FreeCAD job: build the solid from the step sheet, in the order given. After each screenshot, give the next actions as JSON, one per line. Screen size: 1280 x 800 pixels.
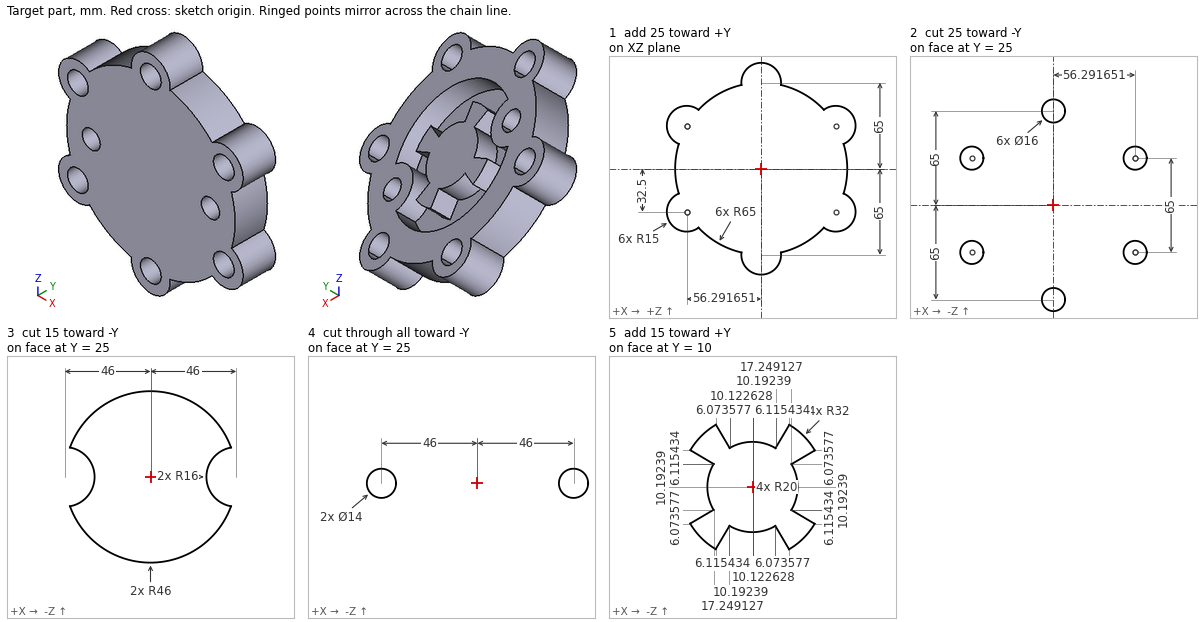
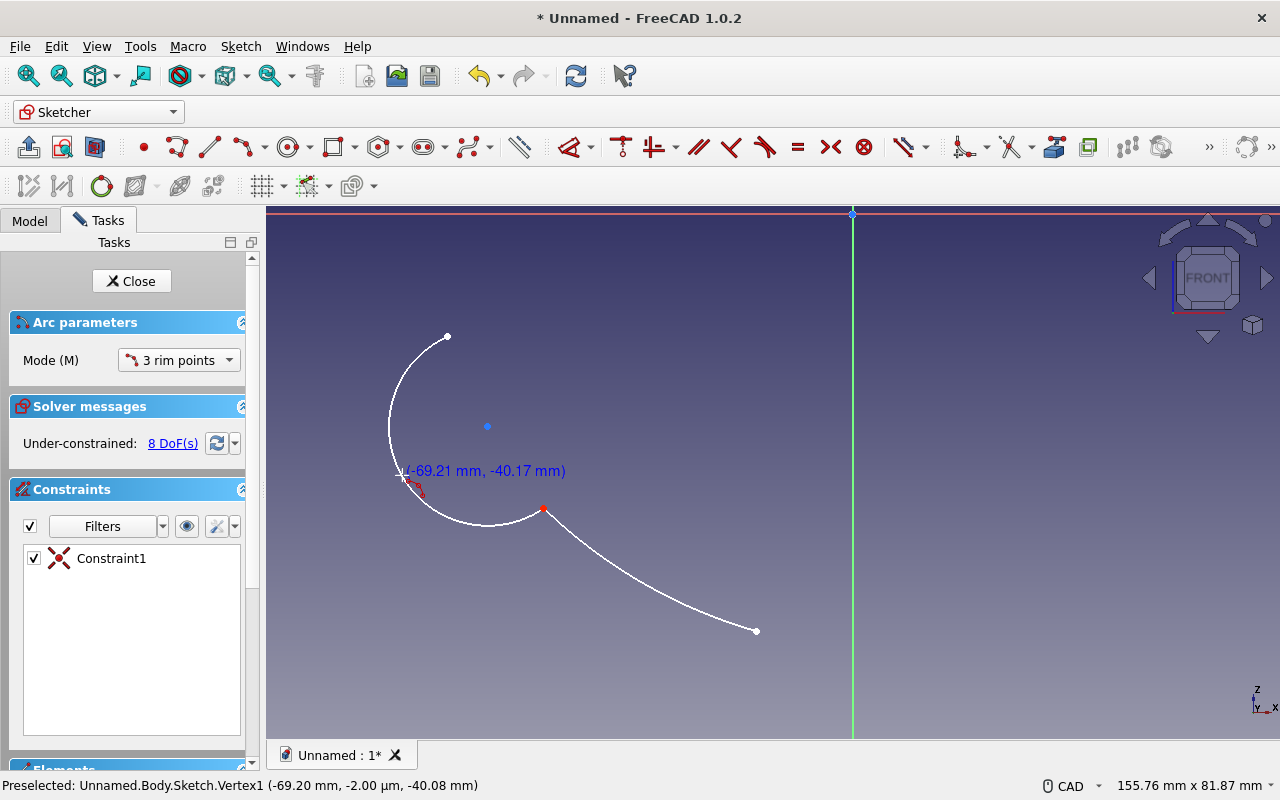
{"action": "left_click", "coordinate": [447, 337]}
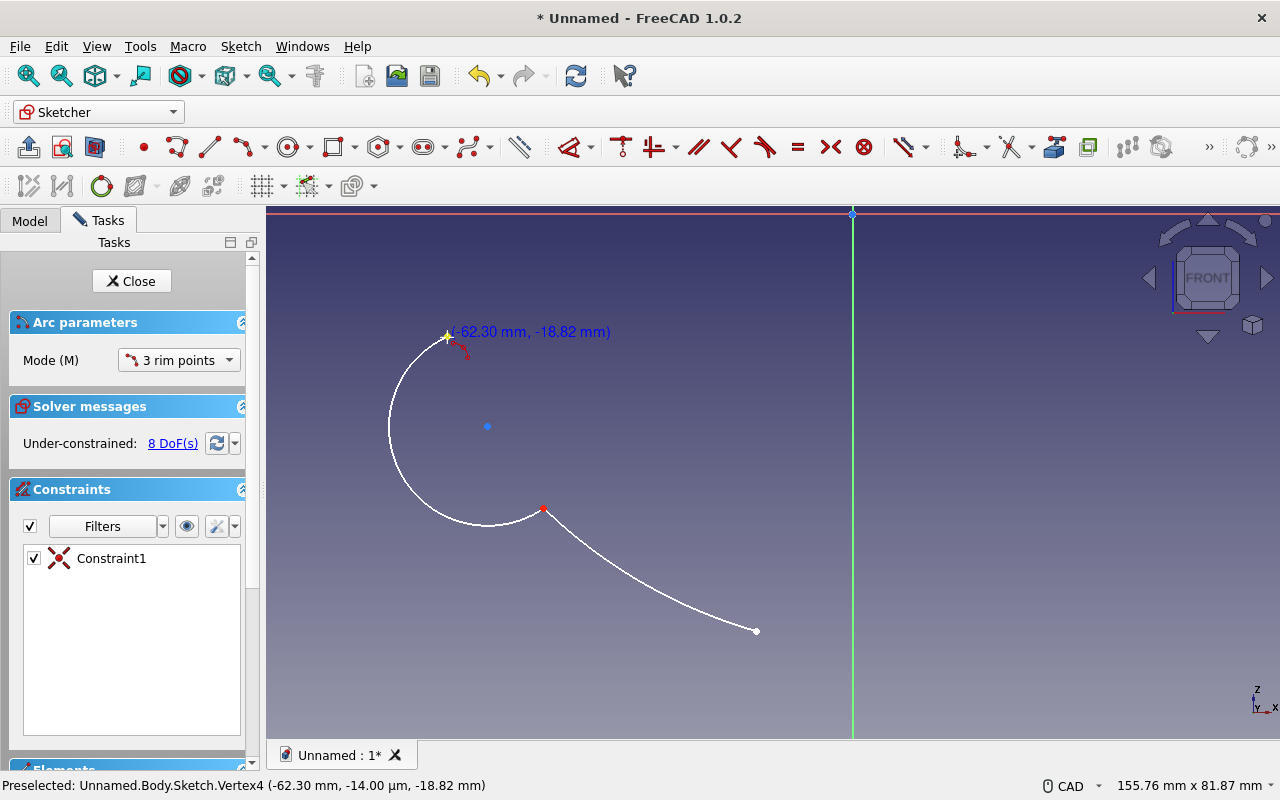
{"action": "scroll", "coordinate": [641, 584], "scroll_direction": "down", "scroll_amount": 6}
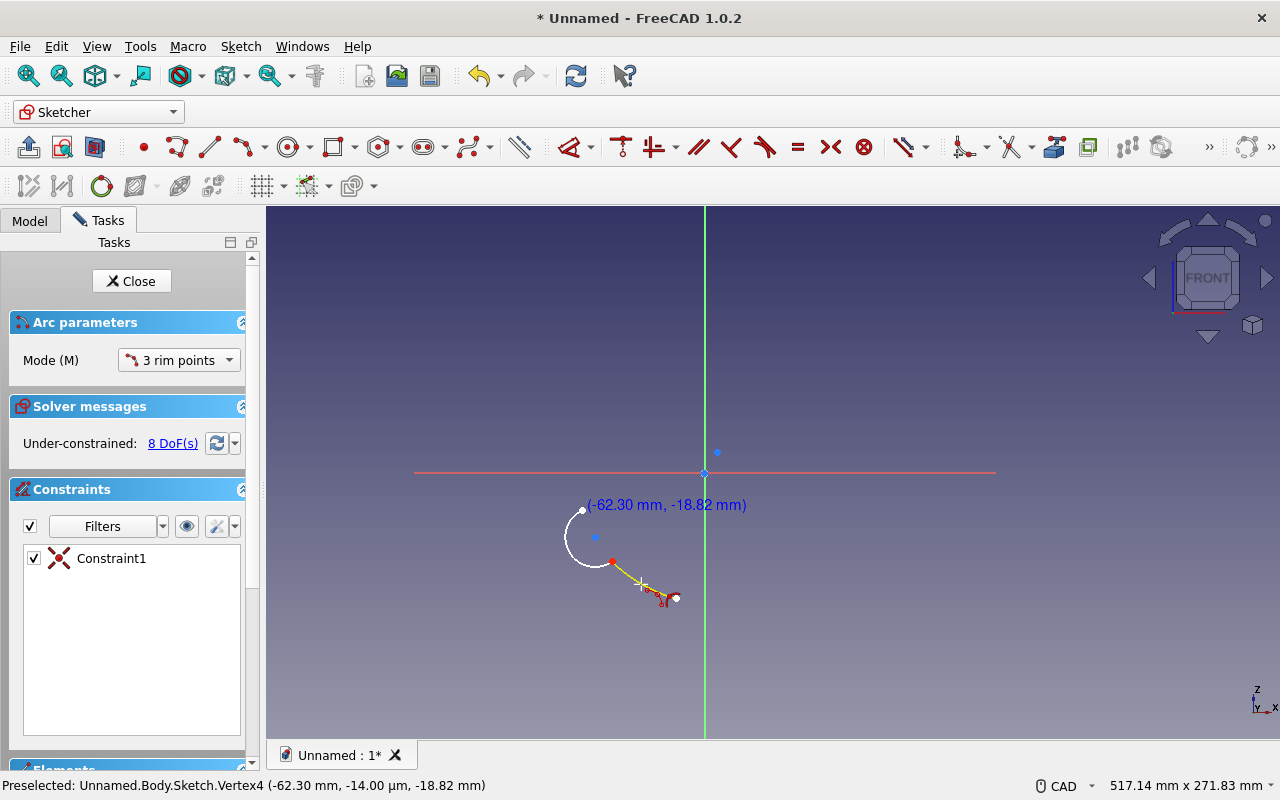
{"action": "left_click", "coordinate": [583, 436]}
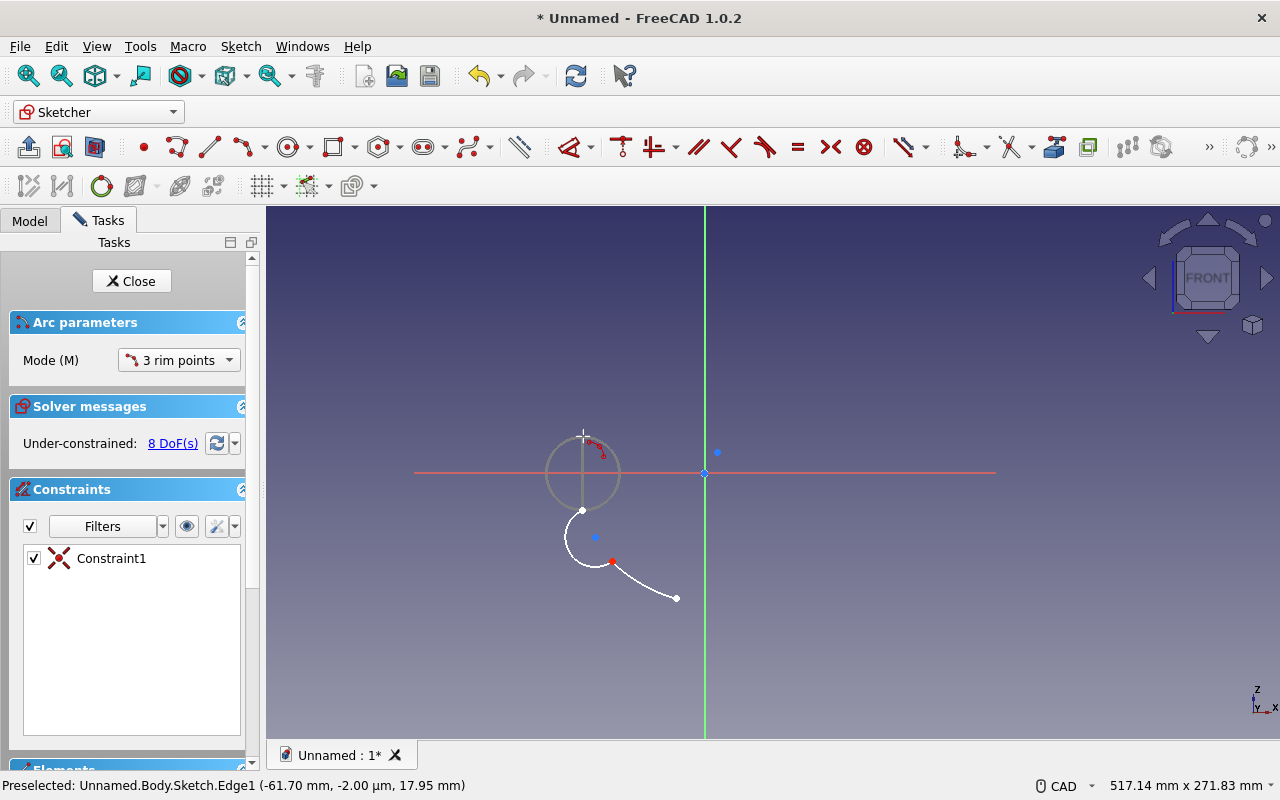
{"action": "scroll", "coordinate": [578, 466], "scroll_direction": "up", "scroll_amount": 6}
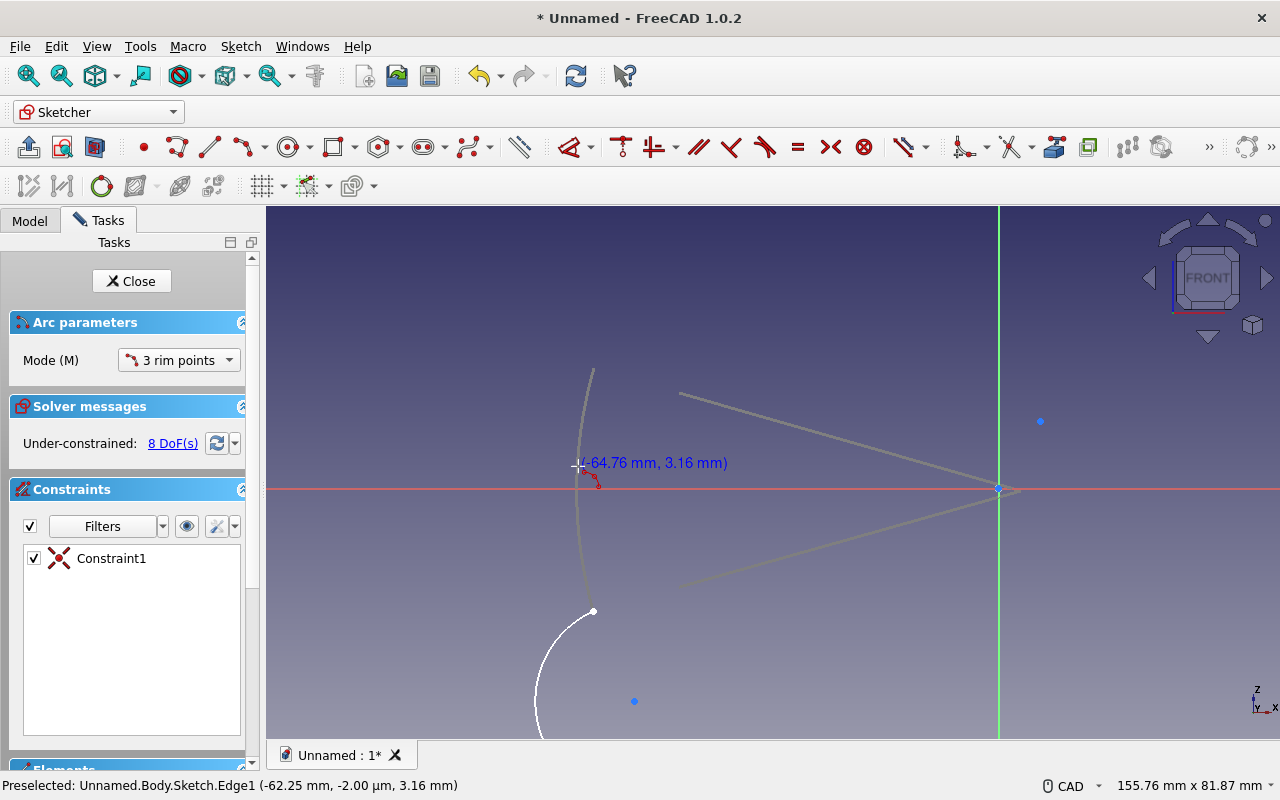
{"action": "left_click", "coordinate": [576, 464]}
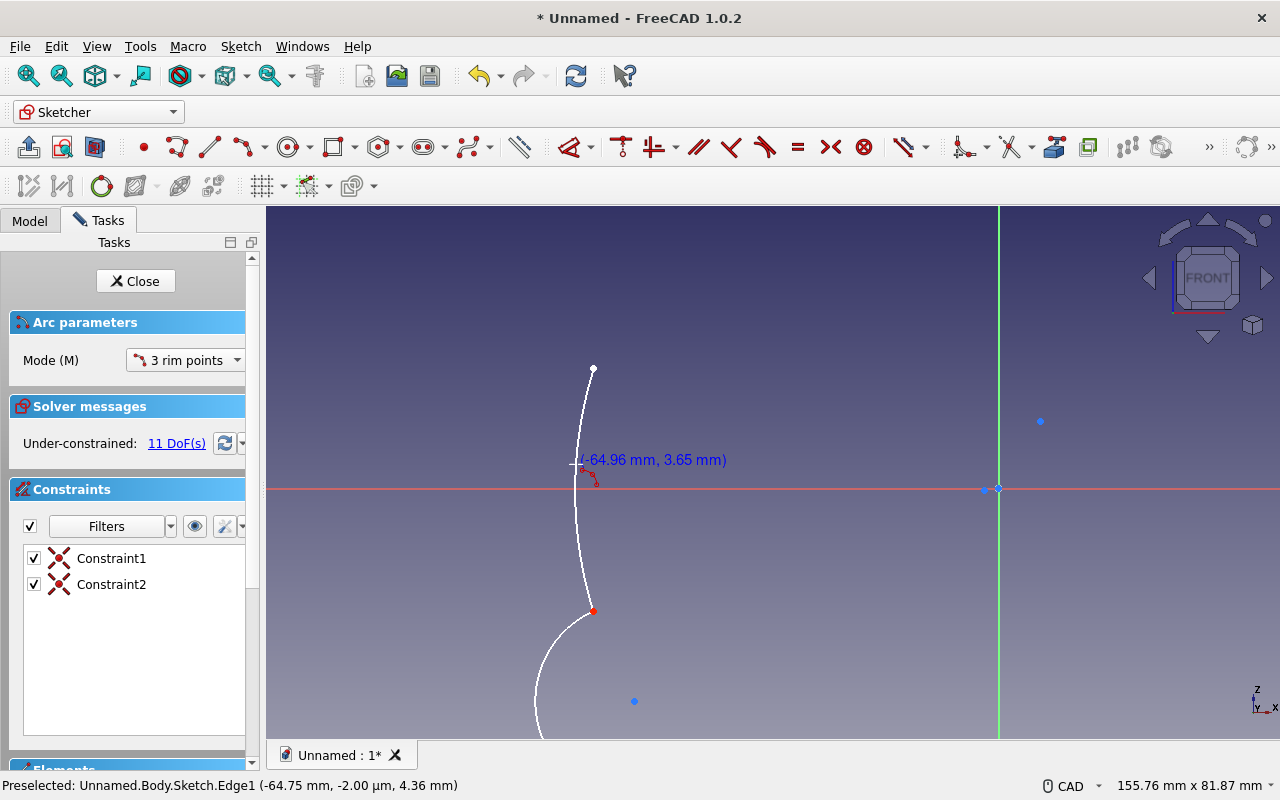
{"action": "left_click", "coordinate": [594, 369]}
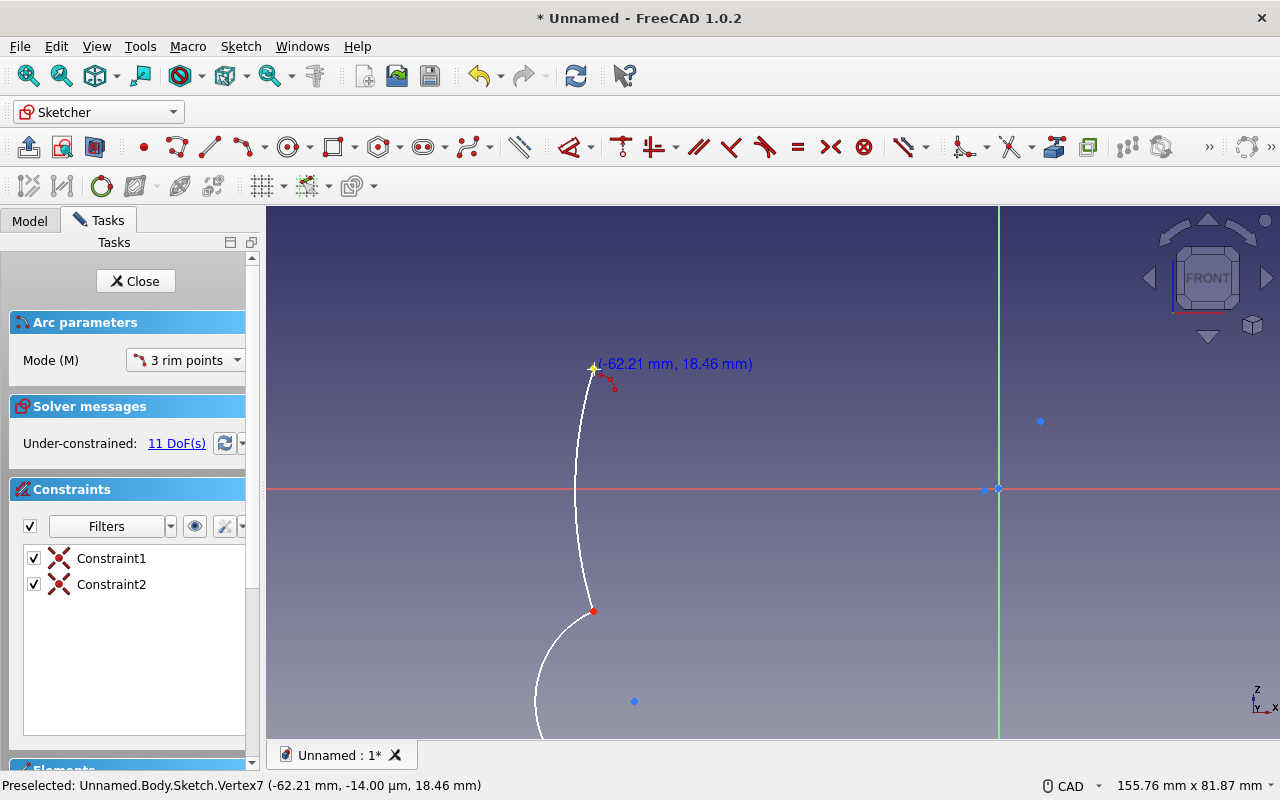
{"action": "scroll", "coordinate": [578, 465], "scroll_direction": "down", "scroll_amount": 6}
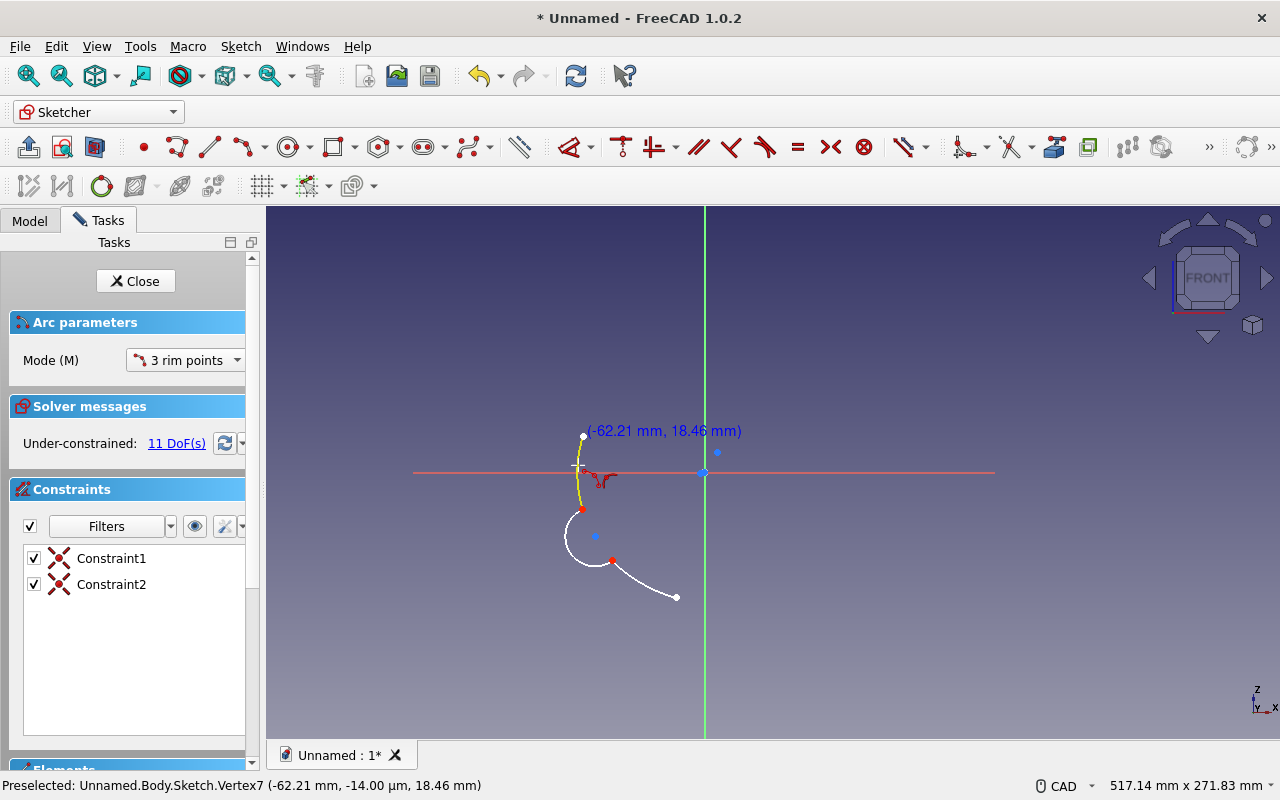
{"action": "left_click", "coordinate": [612, 385]}
{"action": "left_click", "coordinate": [569, 394]}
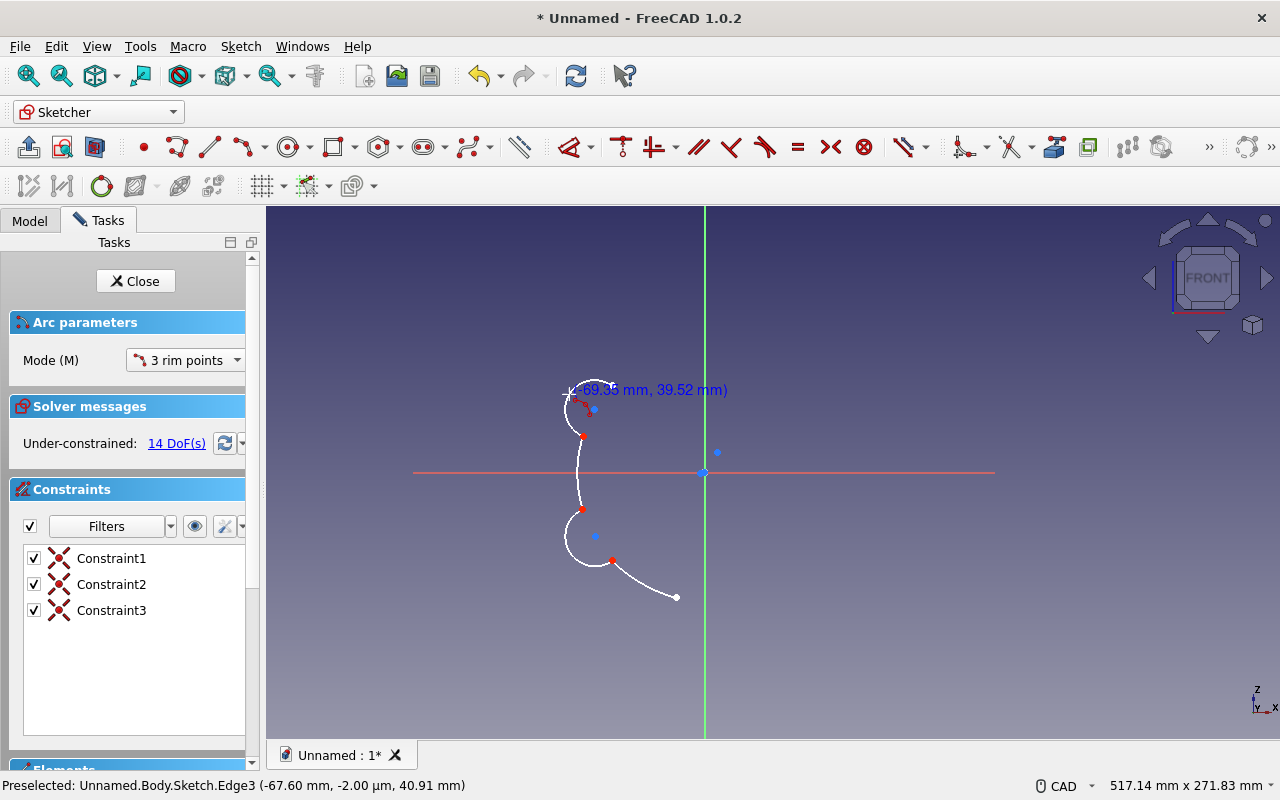
{"action": "left_click", "coordinate": [612, 386]}
{"action": "left_click", "coordinate": [676, 348]}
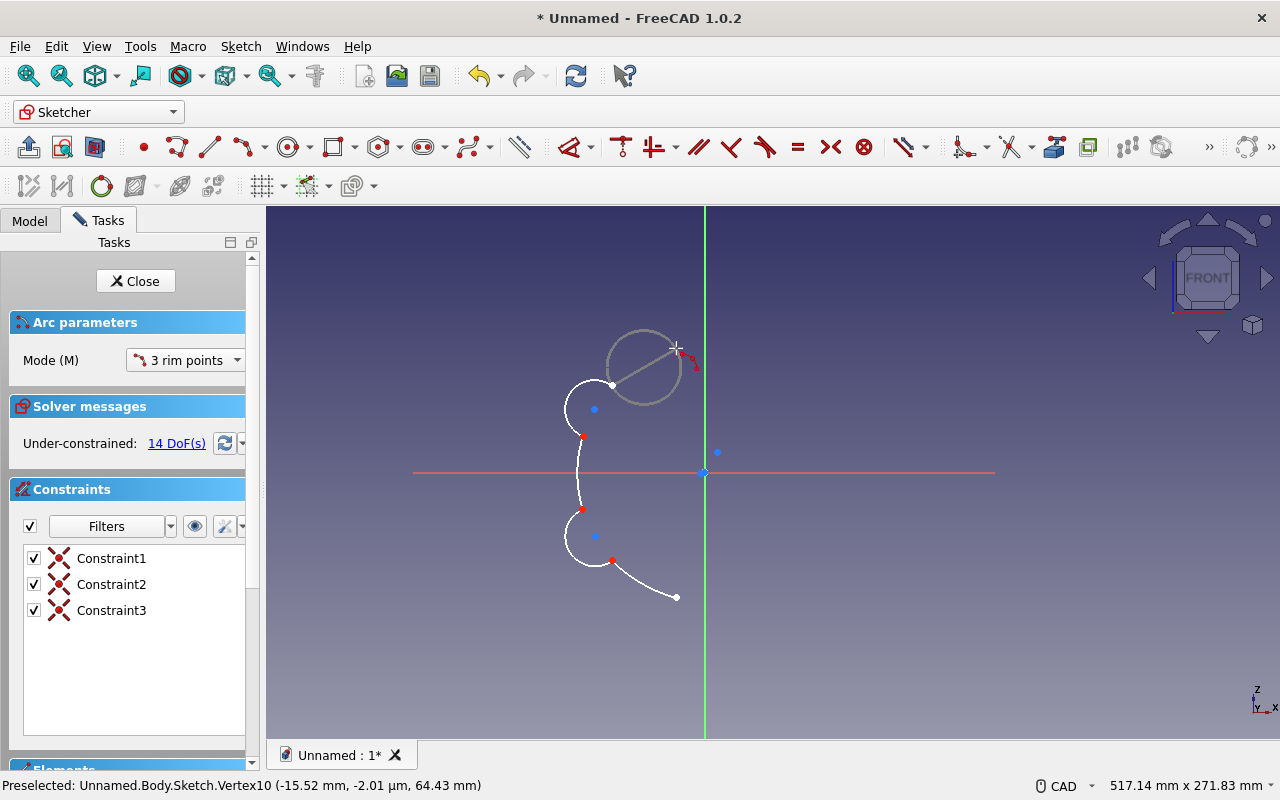
{"action": "scroll", "coordinate": [641, 362], "scroll_direction": "up", "scroll_amount": 6}